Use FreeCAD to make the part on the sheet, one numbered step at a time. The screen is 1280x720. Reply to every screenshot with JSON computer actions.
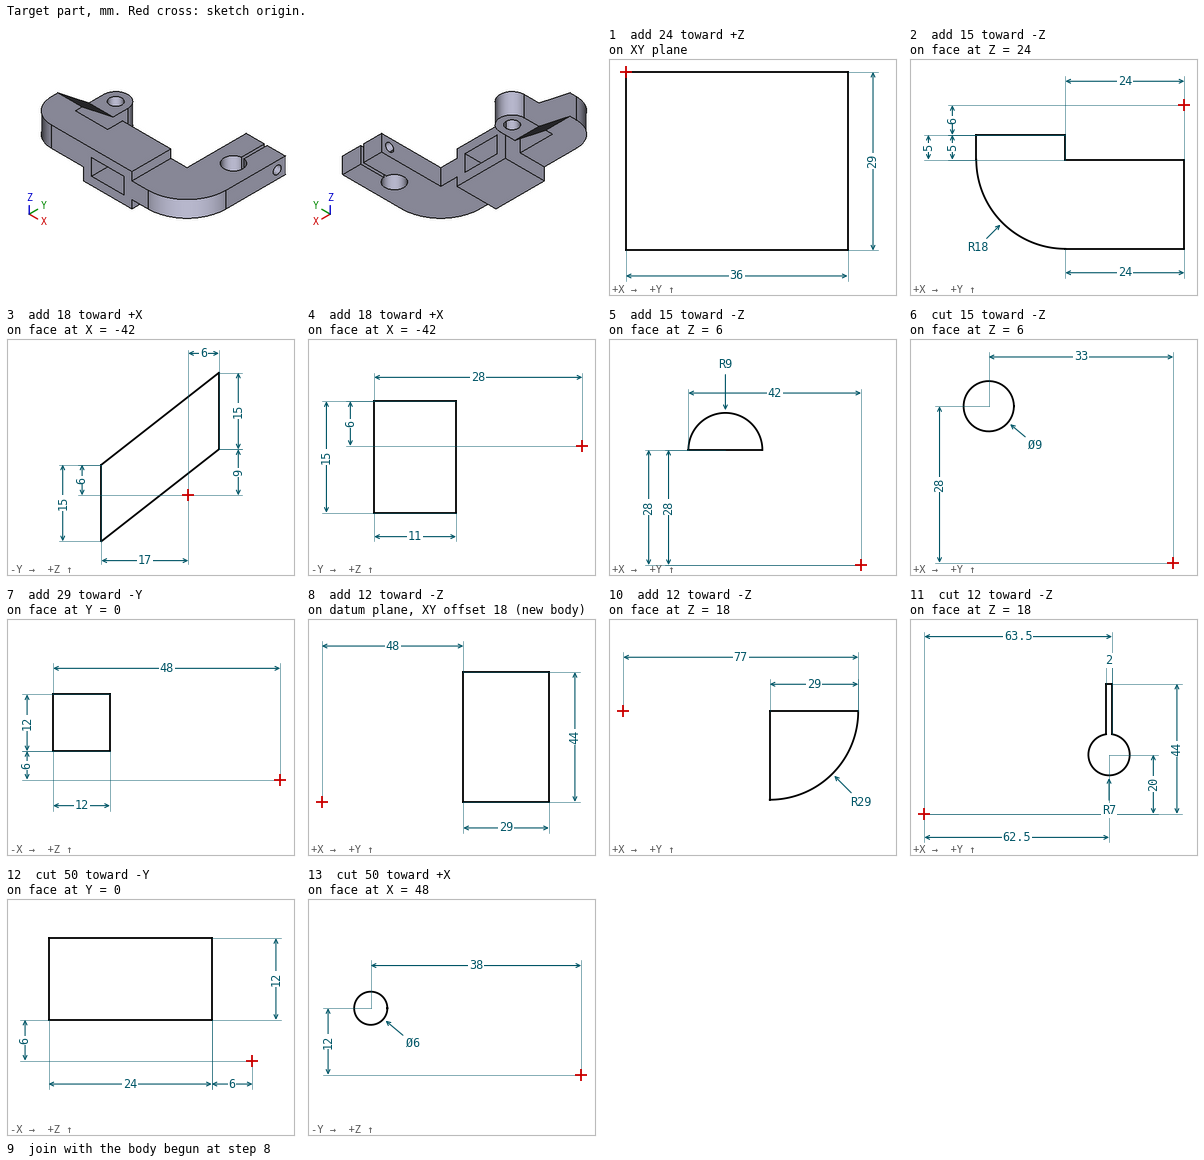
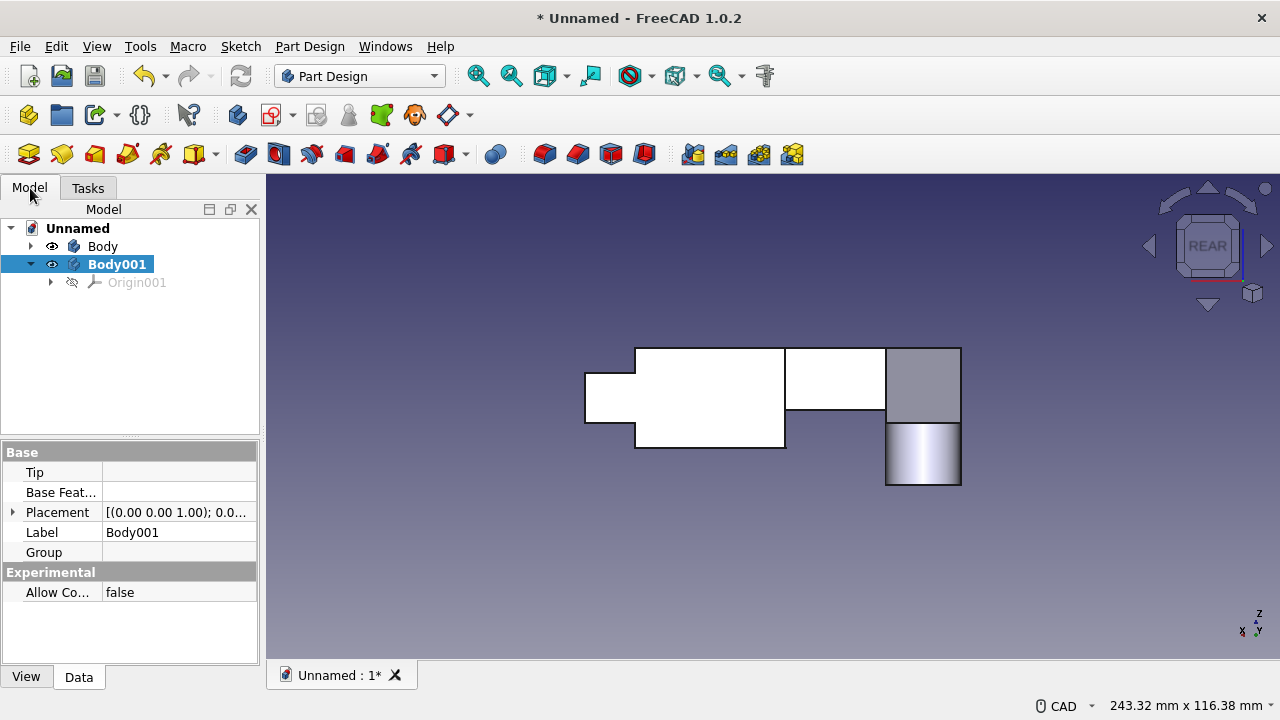
{"action": "left_click", "coordinate": [51, 282]}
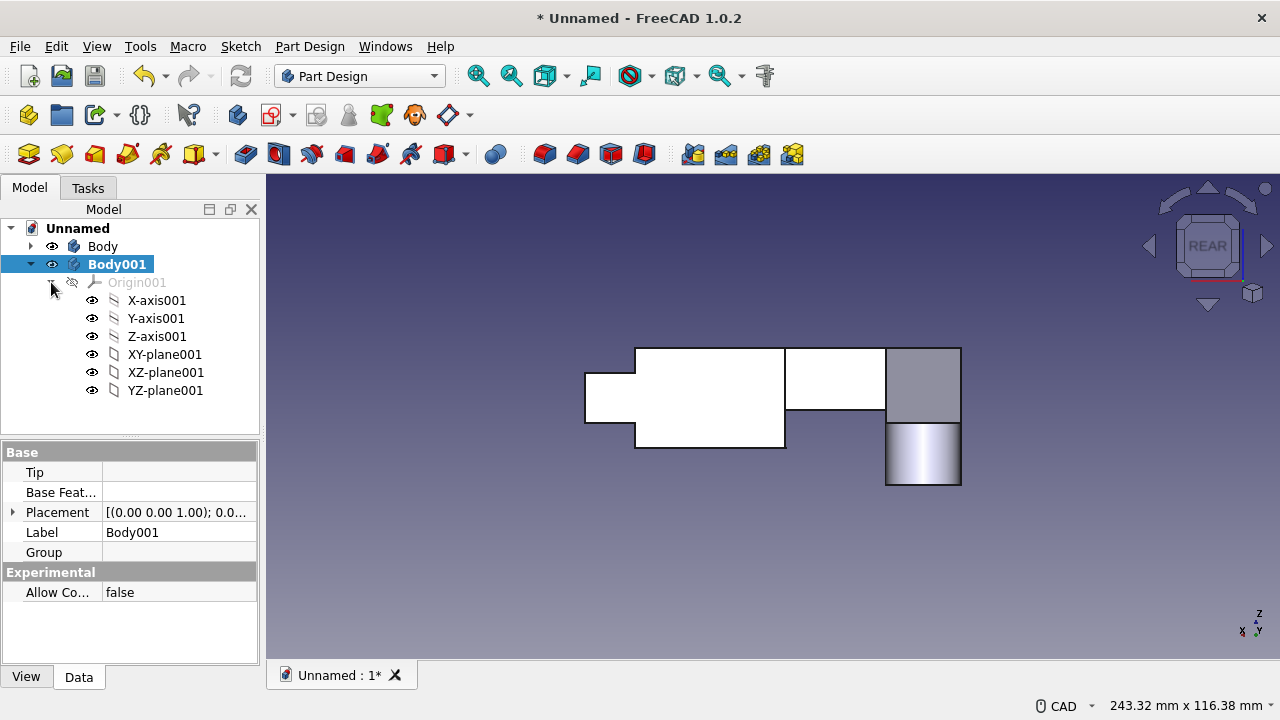
{"action": "left_click", "coordinate": [137, 354]}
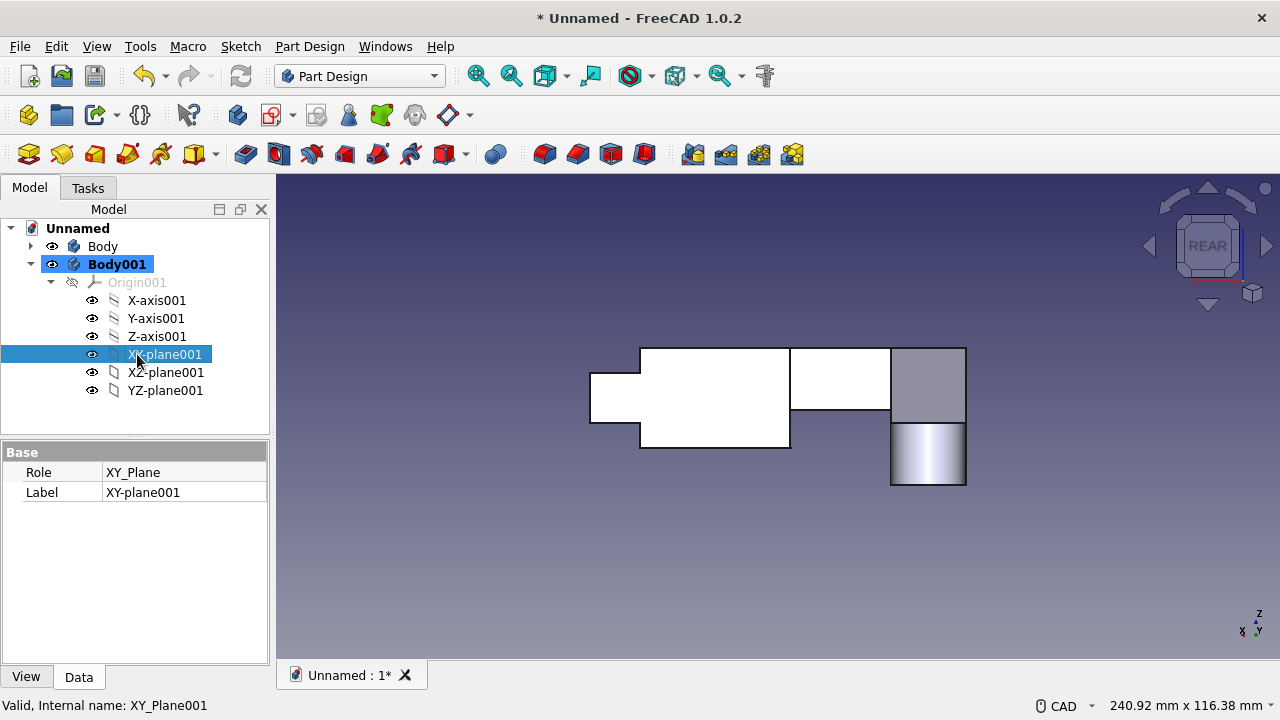
{"action": "left_click", "coordinate": [448, 116]}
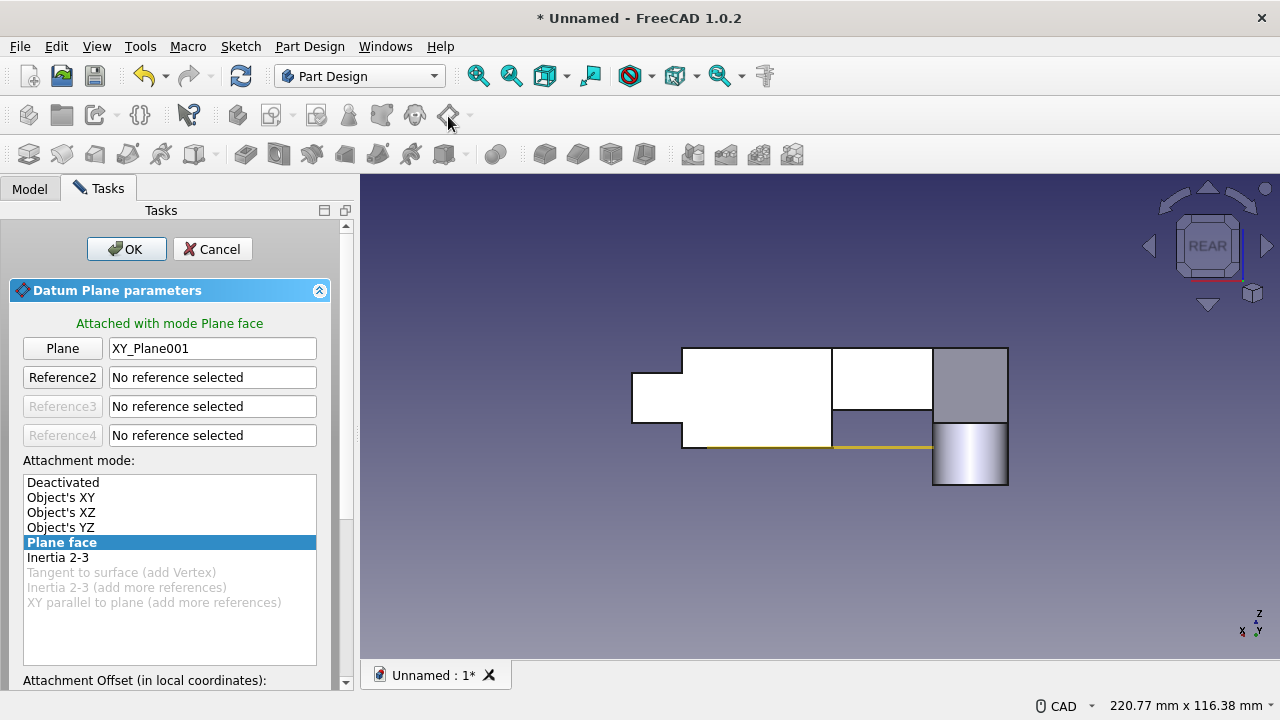
{"action": "scroll", "coordinate": [346, 455], "scroll_direction": "down", "scroll_amount": 3}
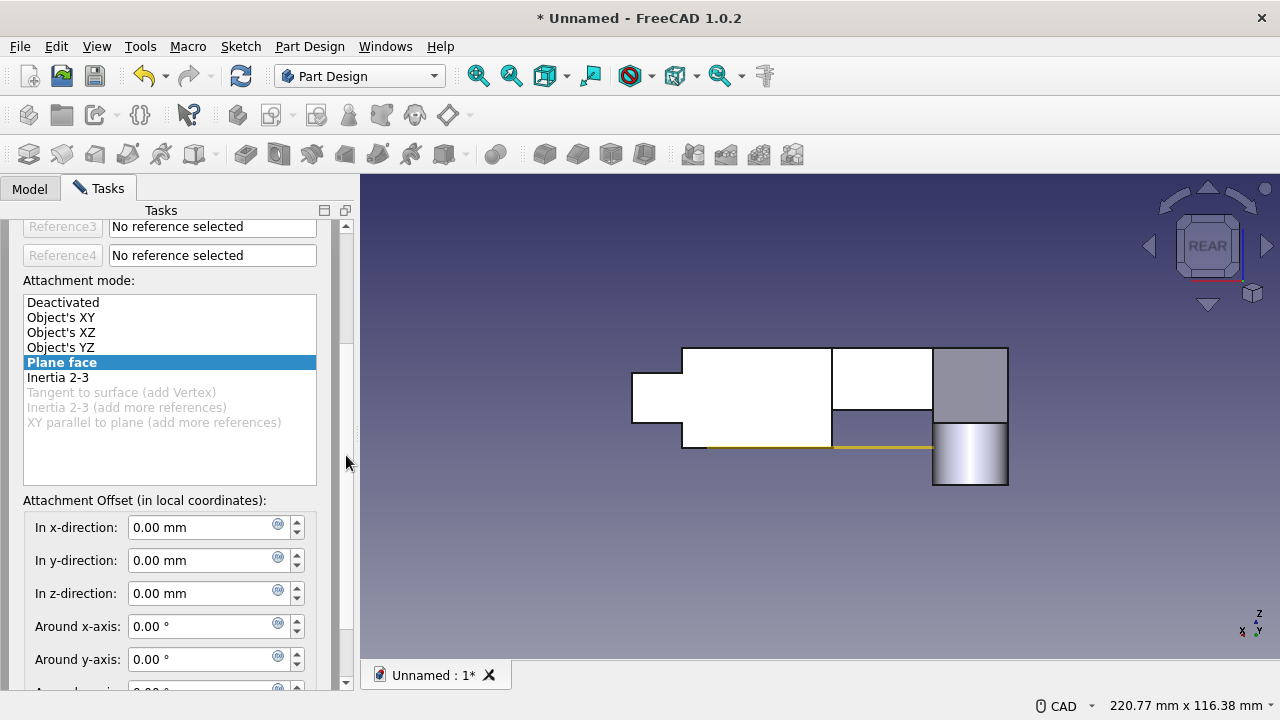
{"action": "triple_click", "coordinate": [210, 594]}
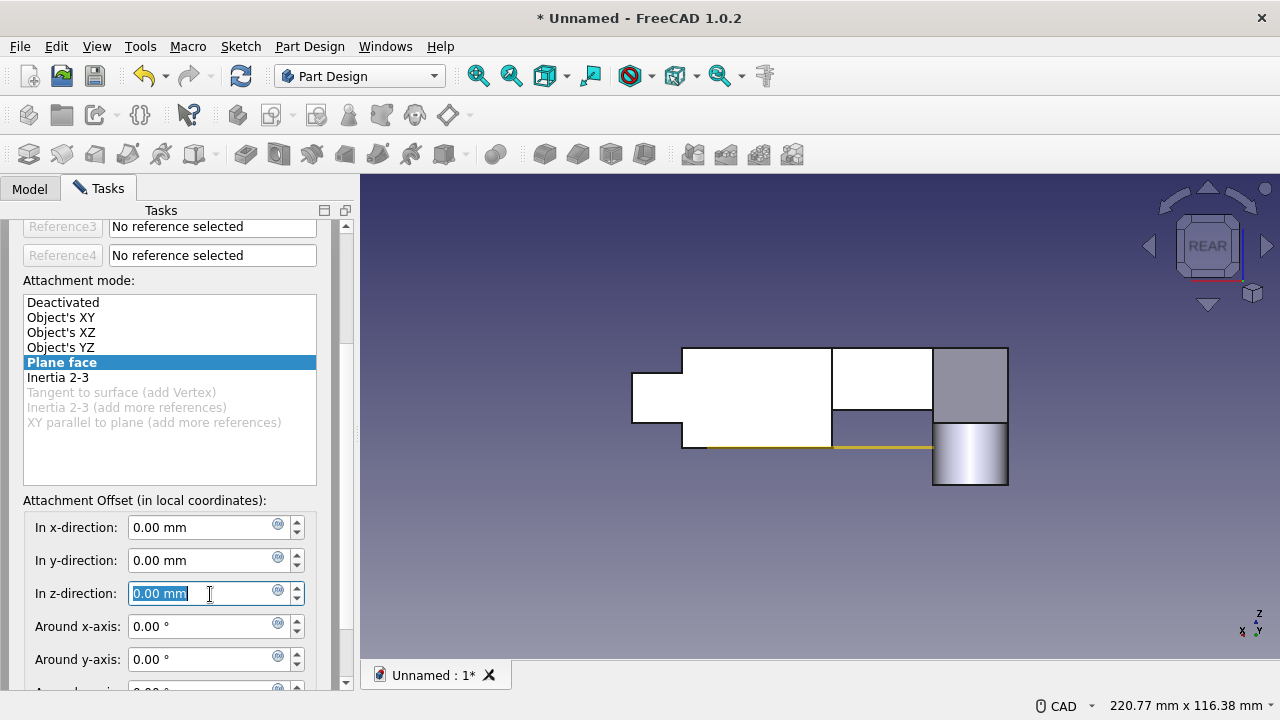
{"action": "type", "text": "18"}
{"action": "key", "text": "Tab"}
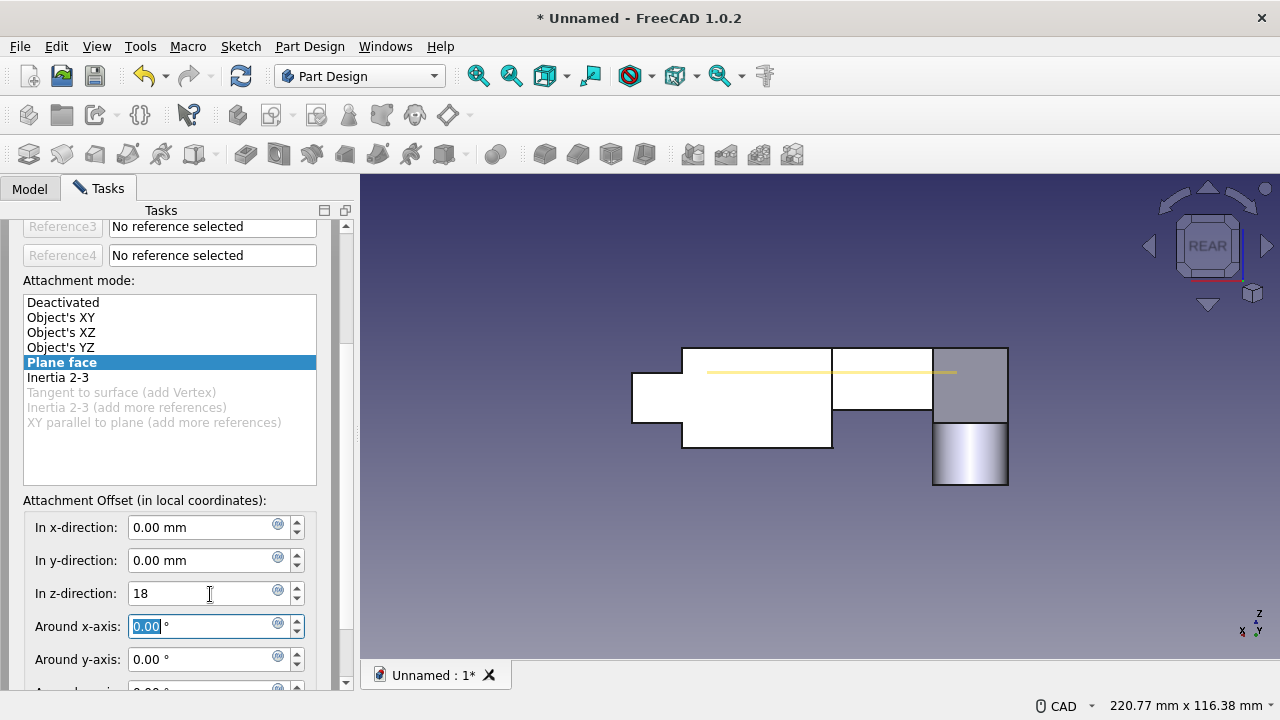
{"action": "scroll", "coordinate": [346, 455], "scroll_direction": "up", "scroll_amount": 4}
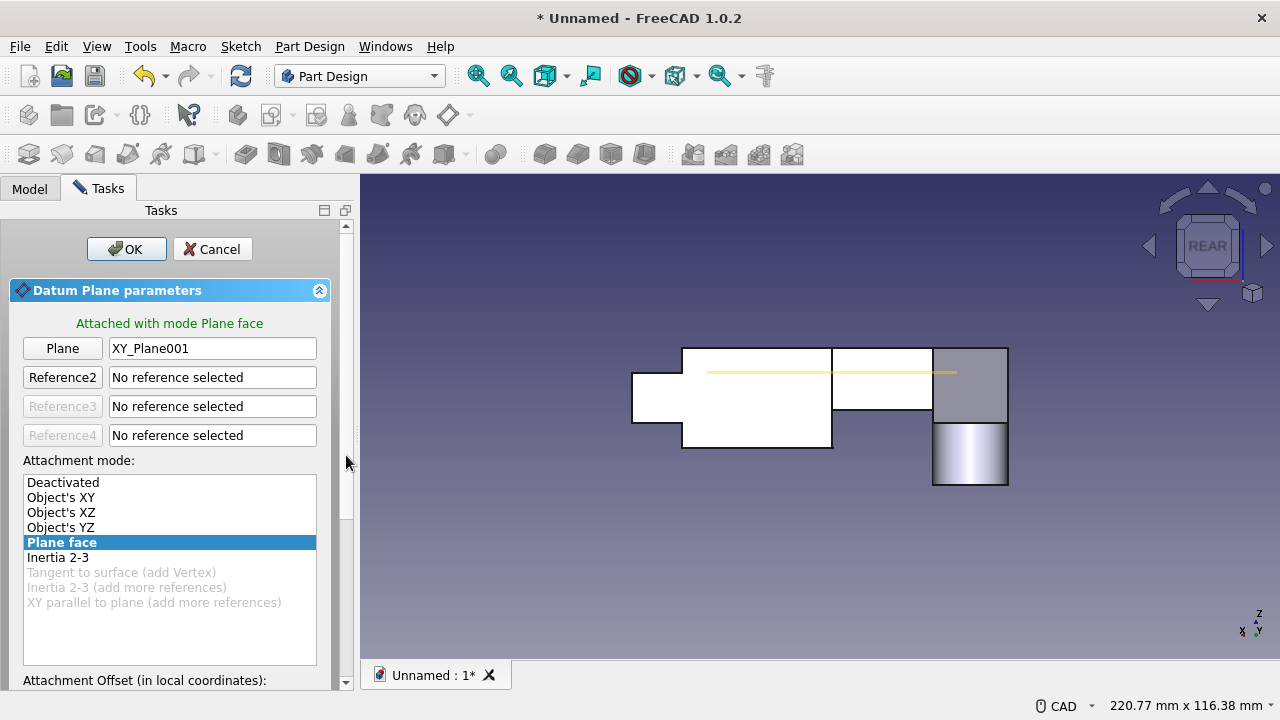
{"action": "left_click", "coordinate": [127, 249]}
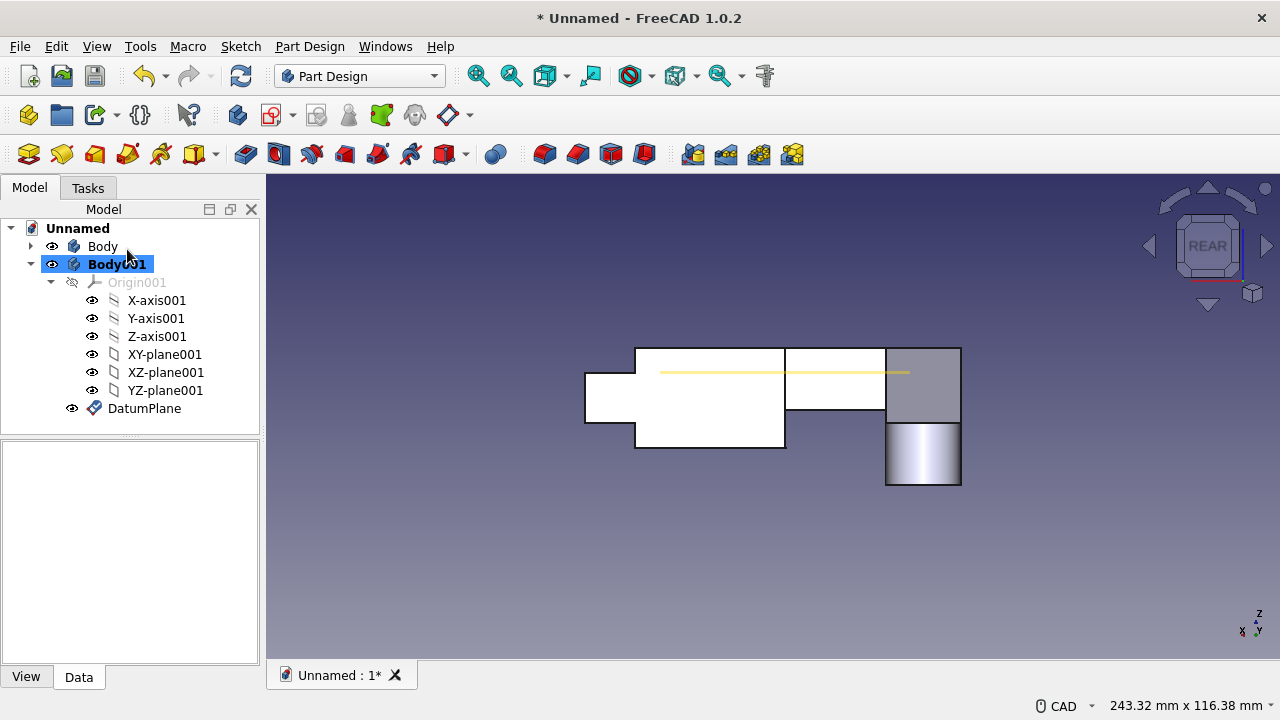
{"action": "left_click", "coordinate": [117, 408]}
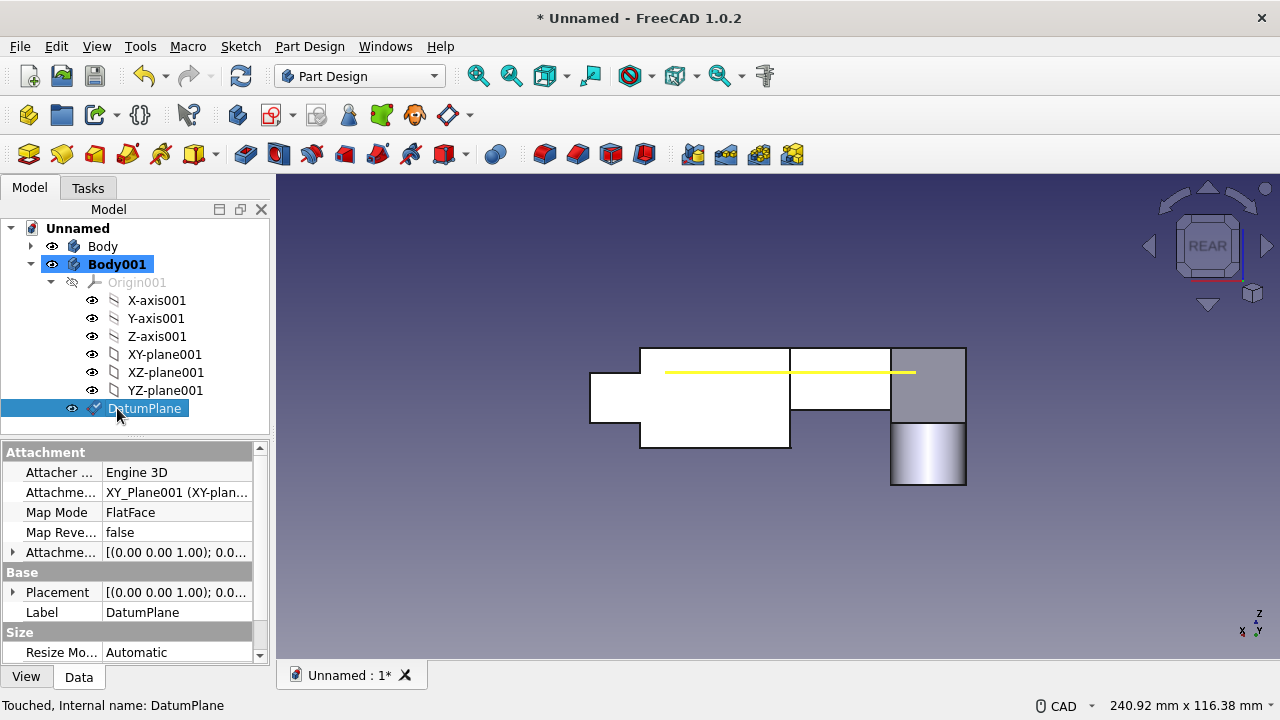
{"action": "left_click", "coordinate": [270, 116]}